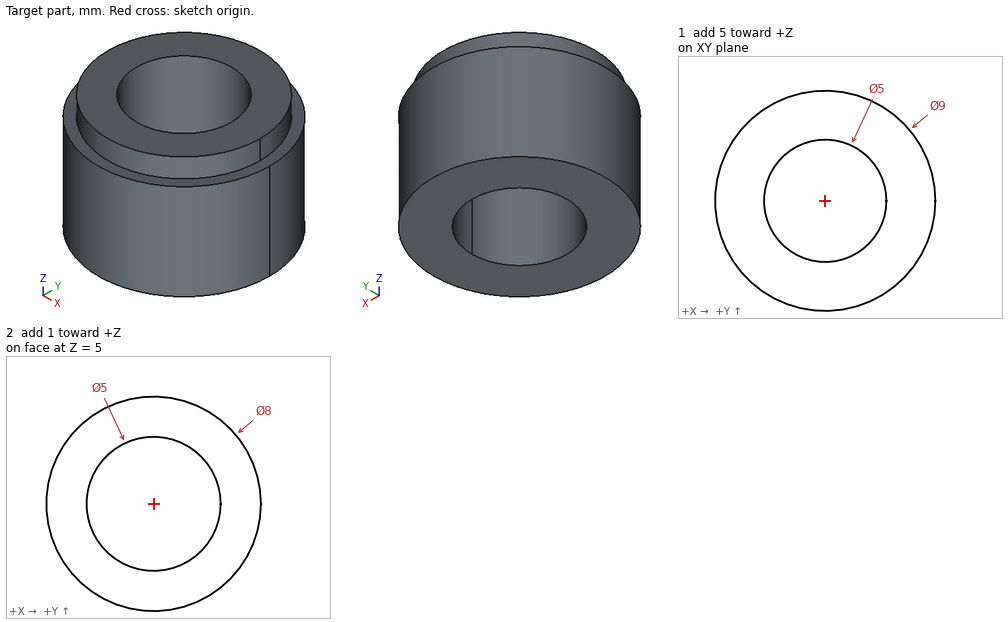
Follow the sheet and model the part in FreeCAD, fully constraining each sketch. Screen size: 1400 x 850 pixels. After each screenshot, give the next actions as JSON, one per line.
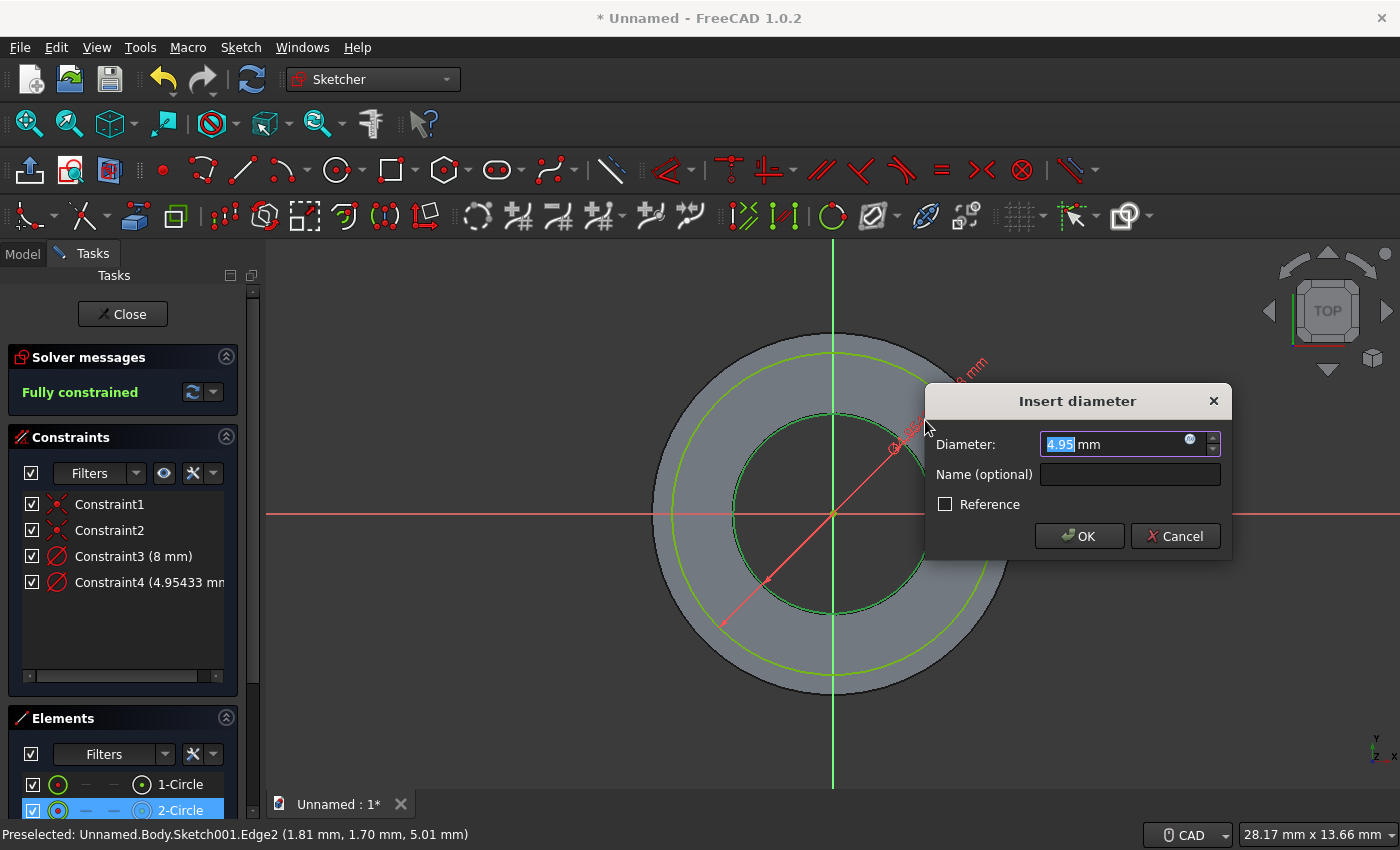
{"action": "type", "text": "5"}
{"action": "key", "text": "Return"}
{"action": "key", "text": "Escape"}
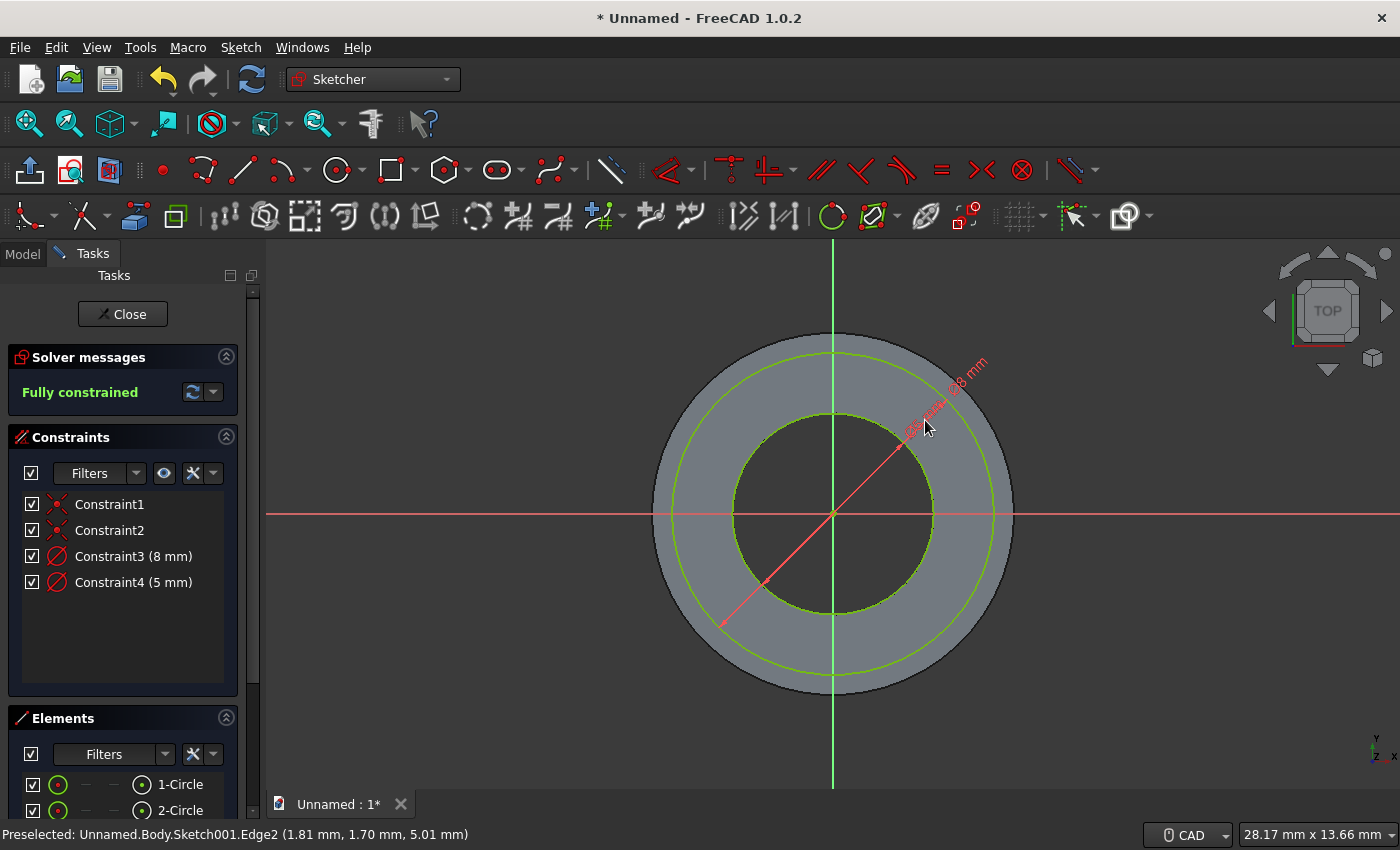
{"action": "left_click", "coordinate": [123, 314]}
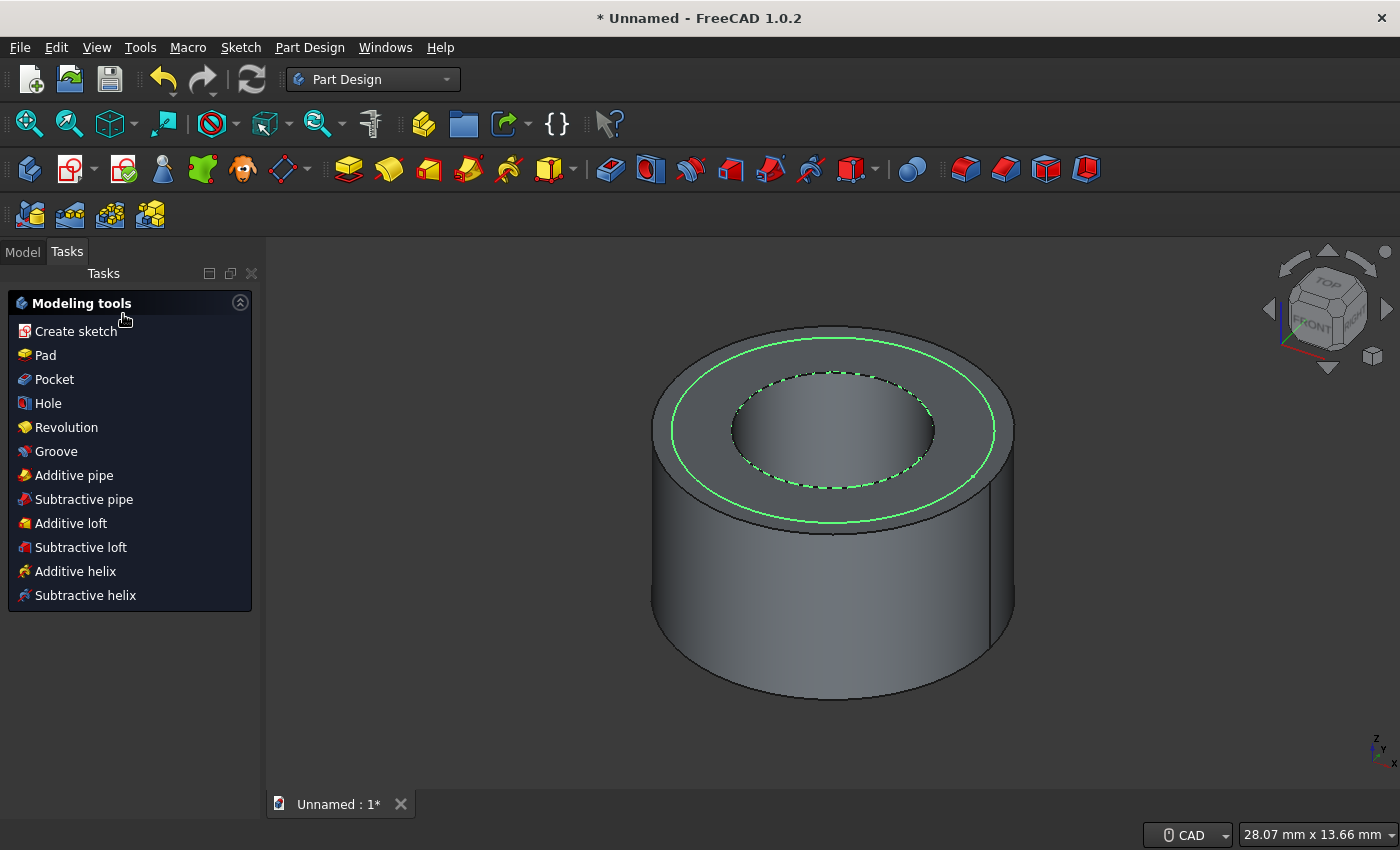
{"action": "left_click", "coordinate": [350, 170]}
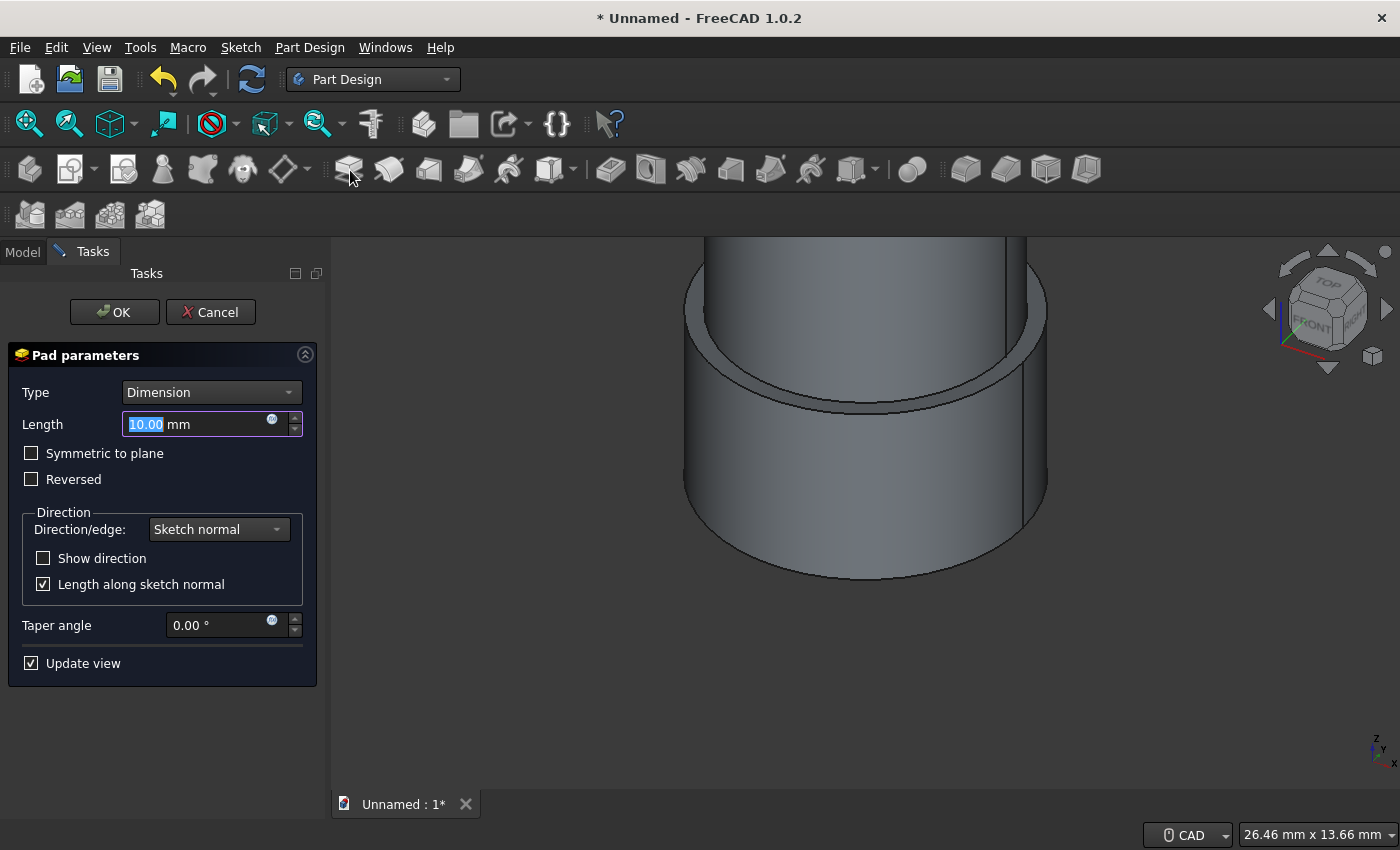
{"action": "type", "text": "1"}
{"action": "key", "text": "Tab"}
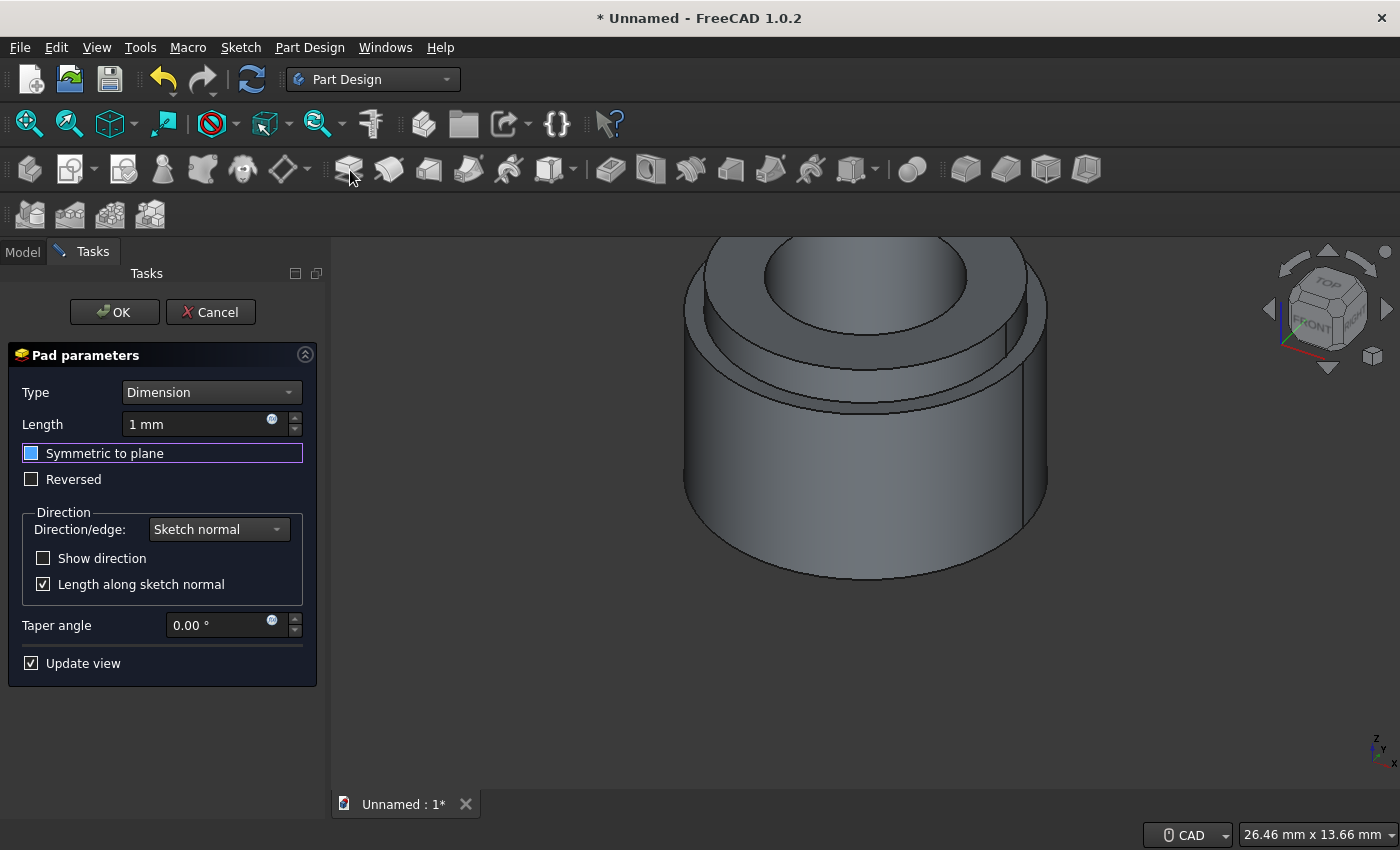
{"action": "left_click", "coordinate": [115, 312]}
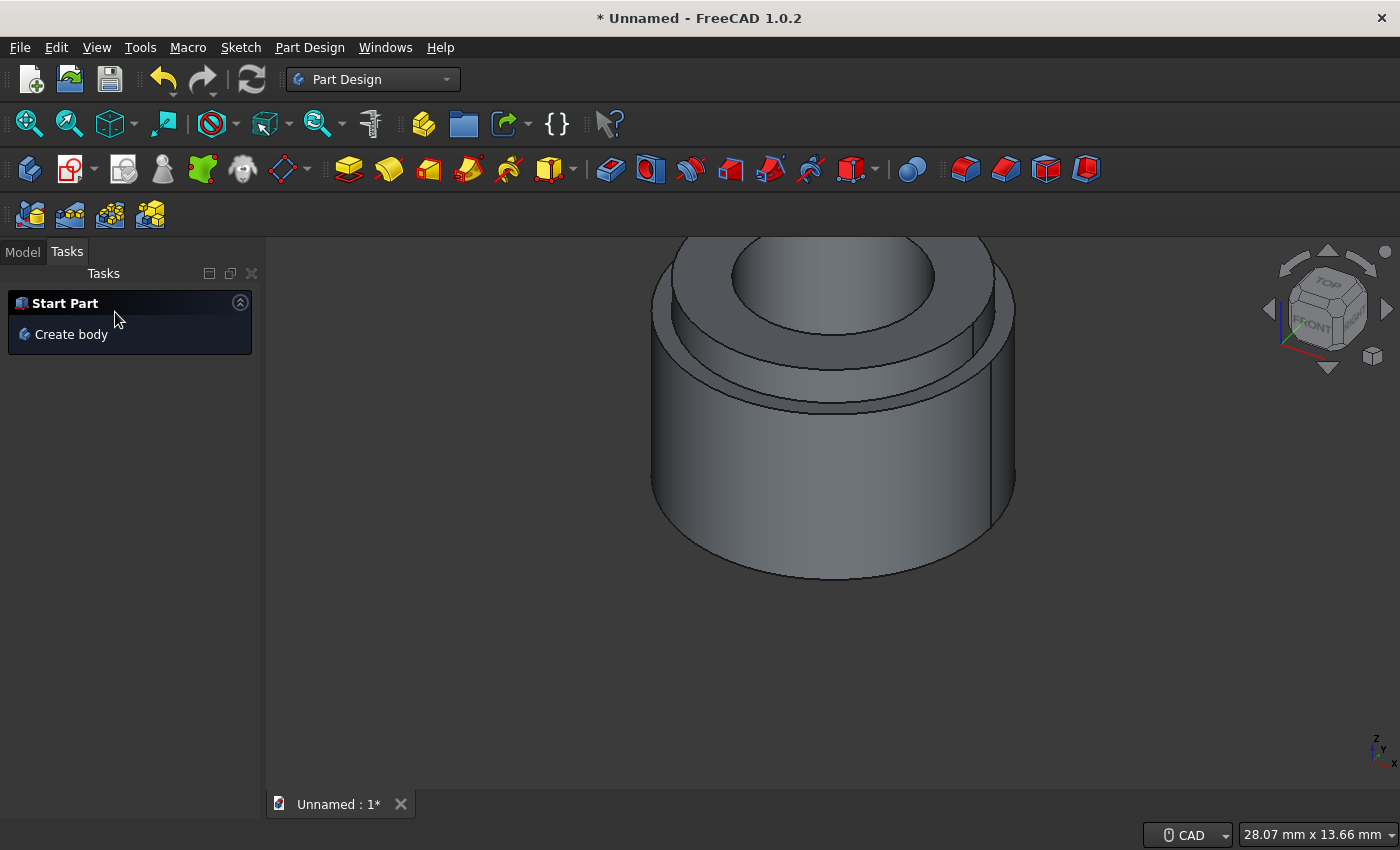
{"action": "key", "text": "0"}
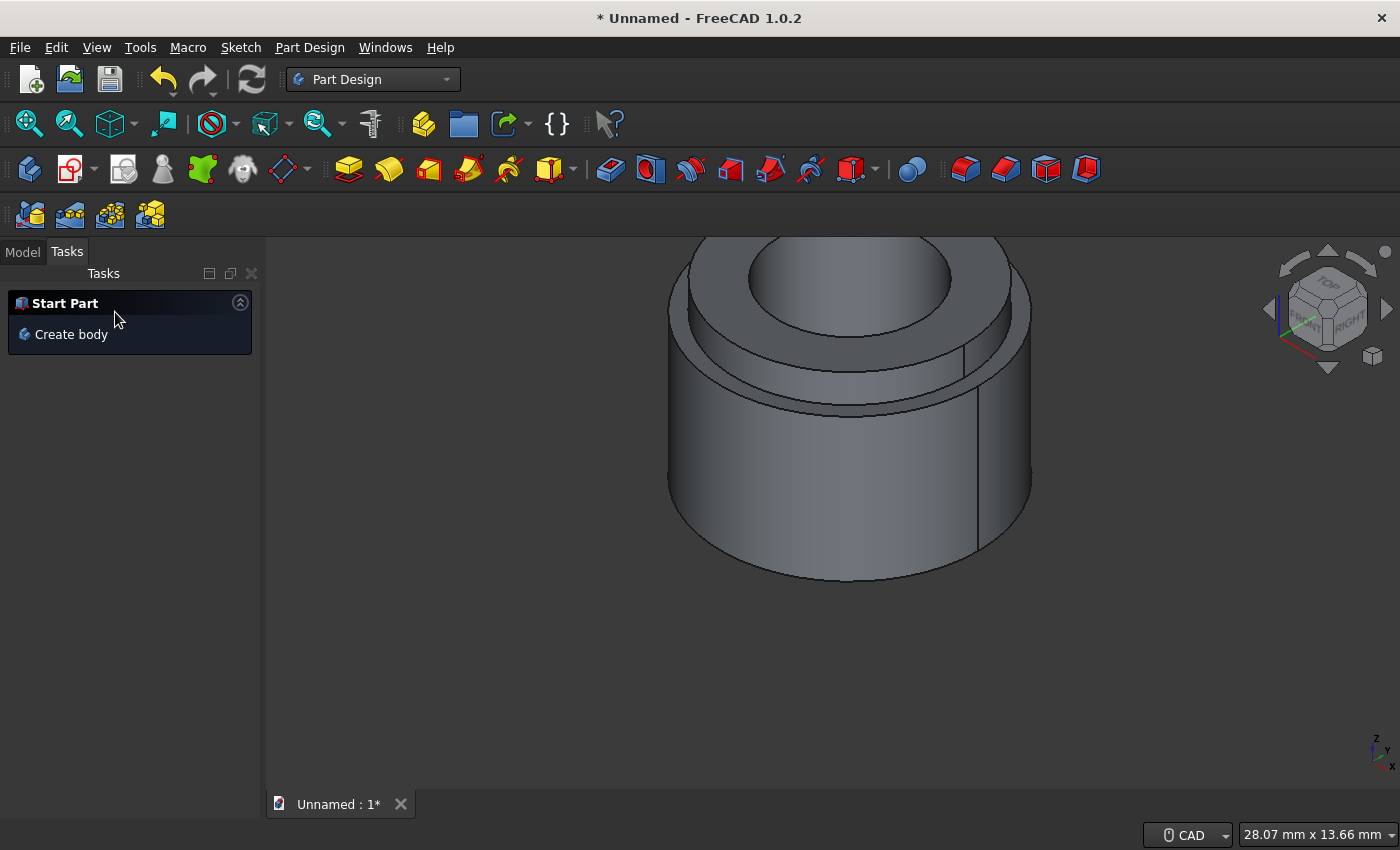
{"action": "left_click", "coordinate": [30, 124]}